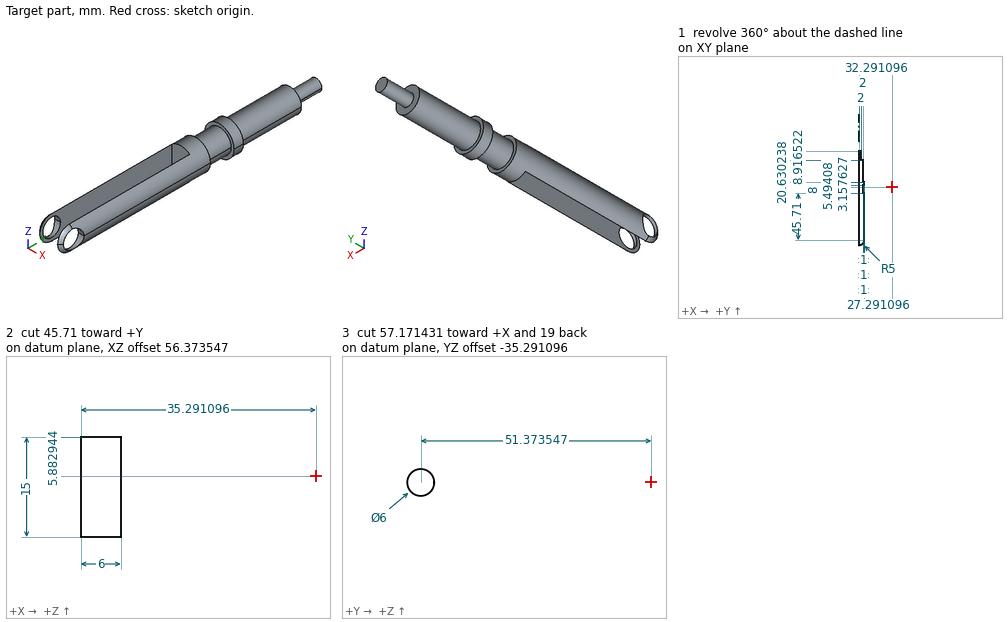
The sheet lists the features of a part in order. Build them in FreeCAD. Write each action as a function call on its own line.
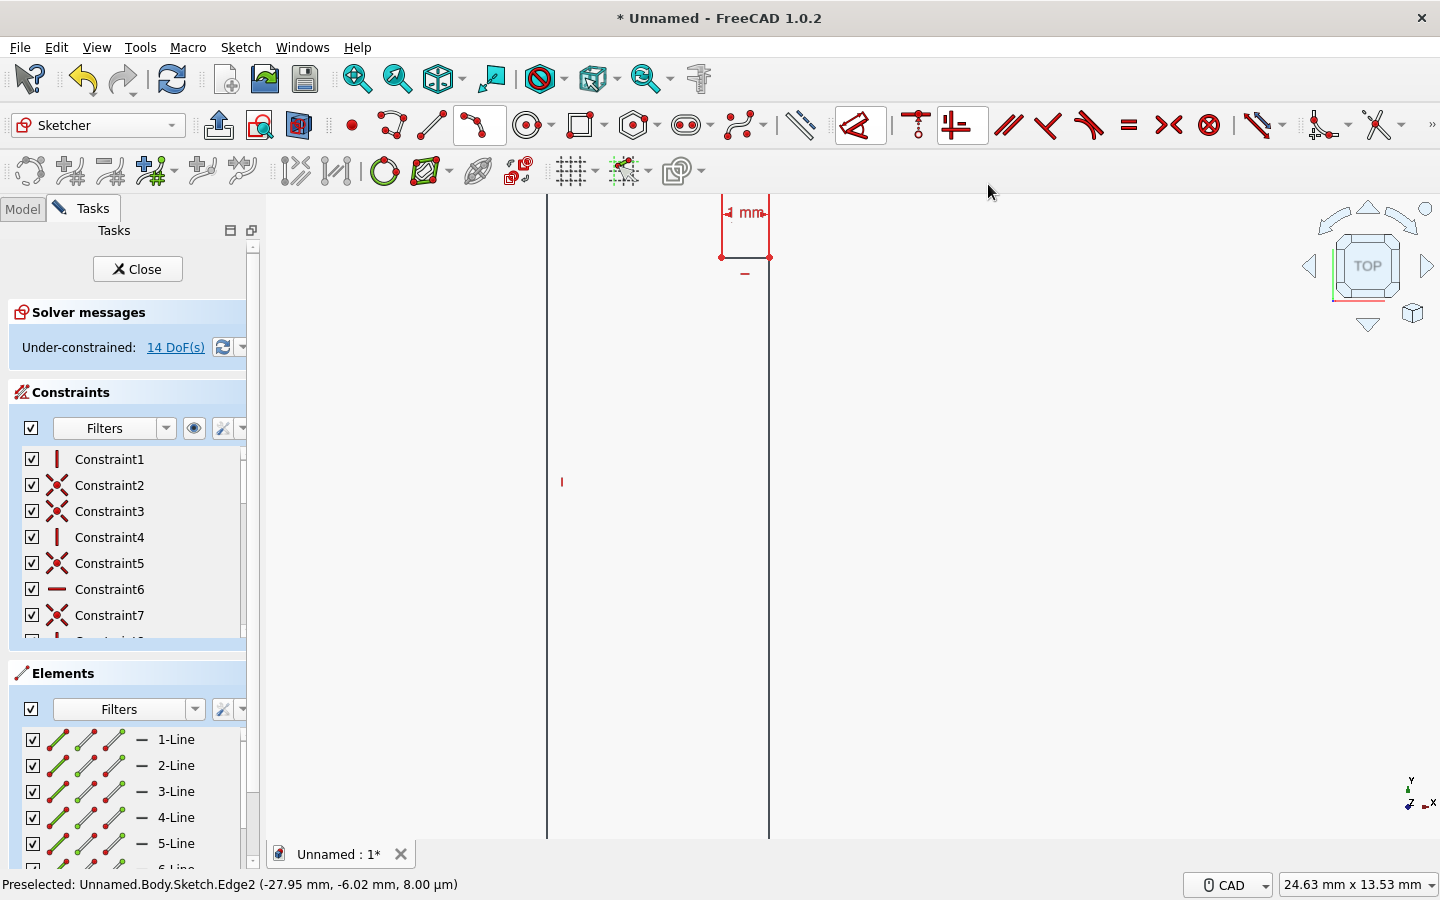
scroll(742, 589, down, 13)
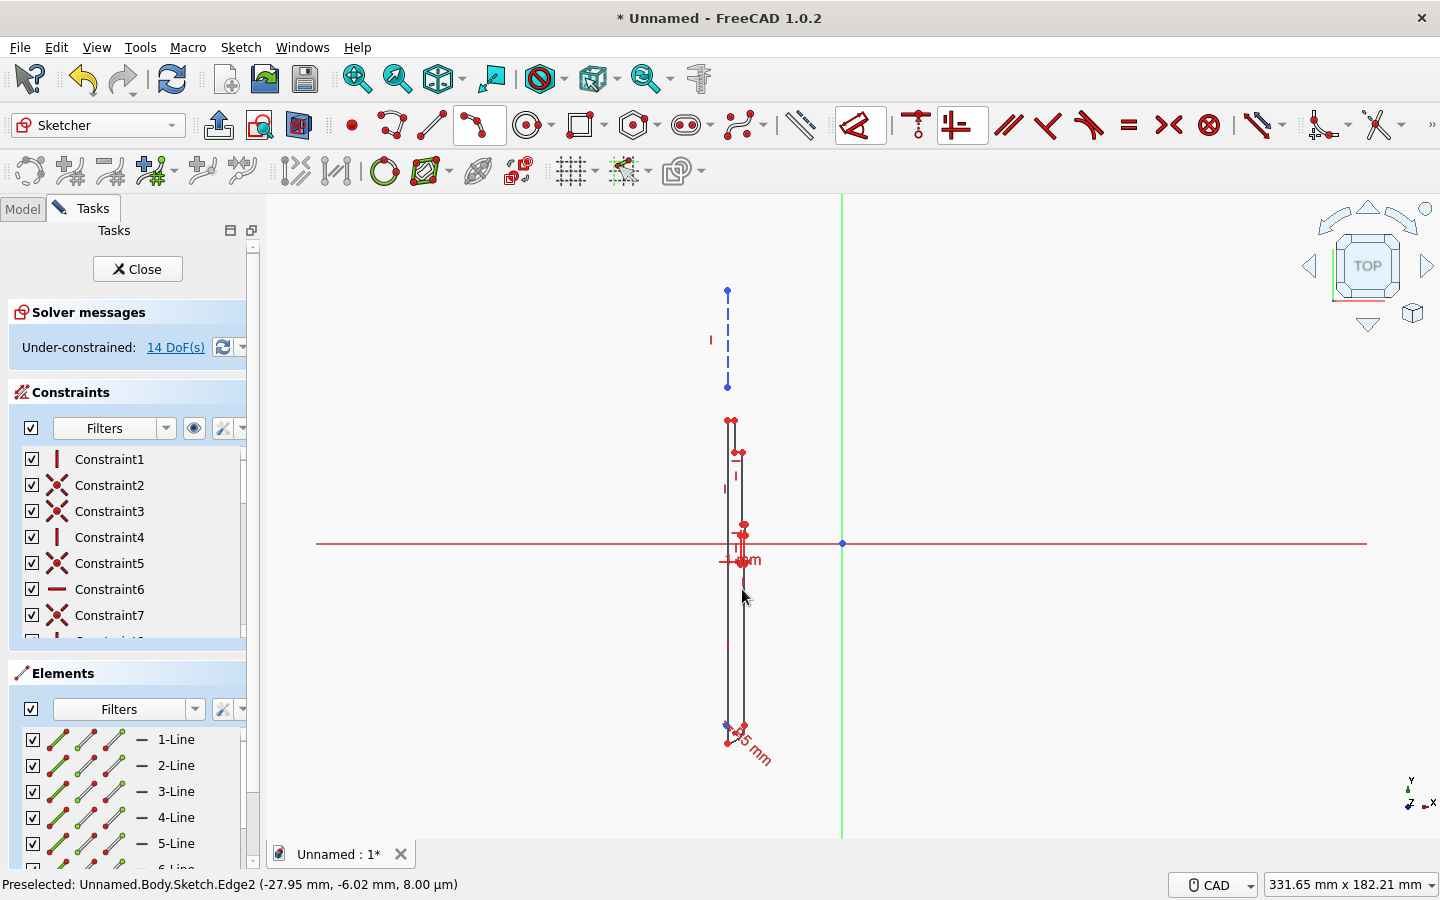
scroll(741, 556, up, 3)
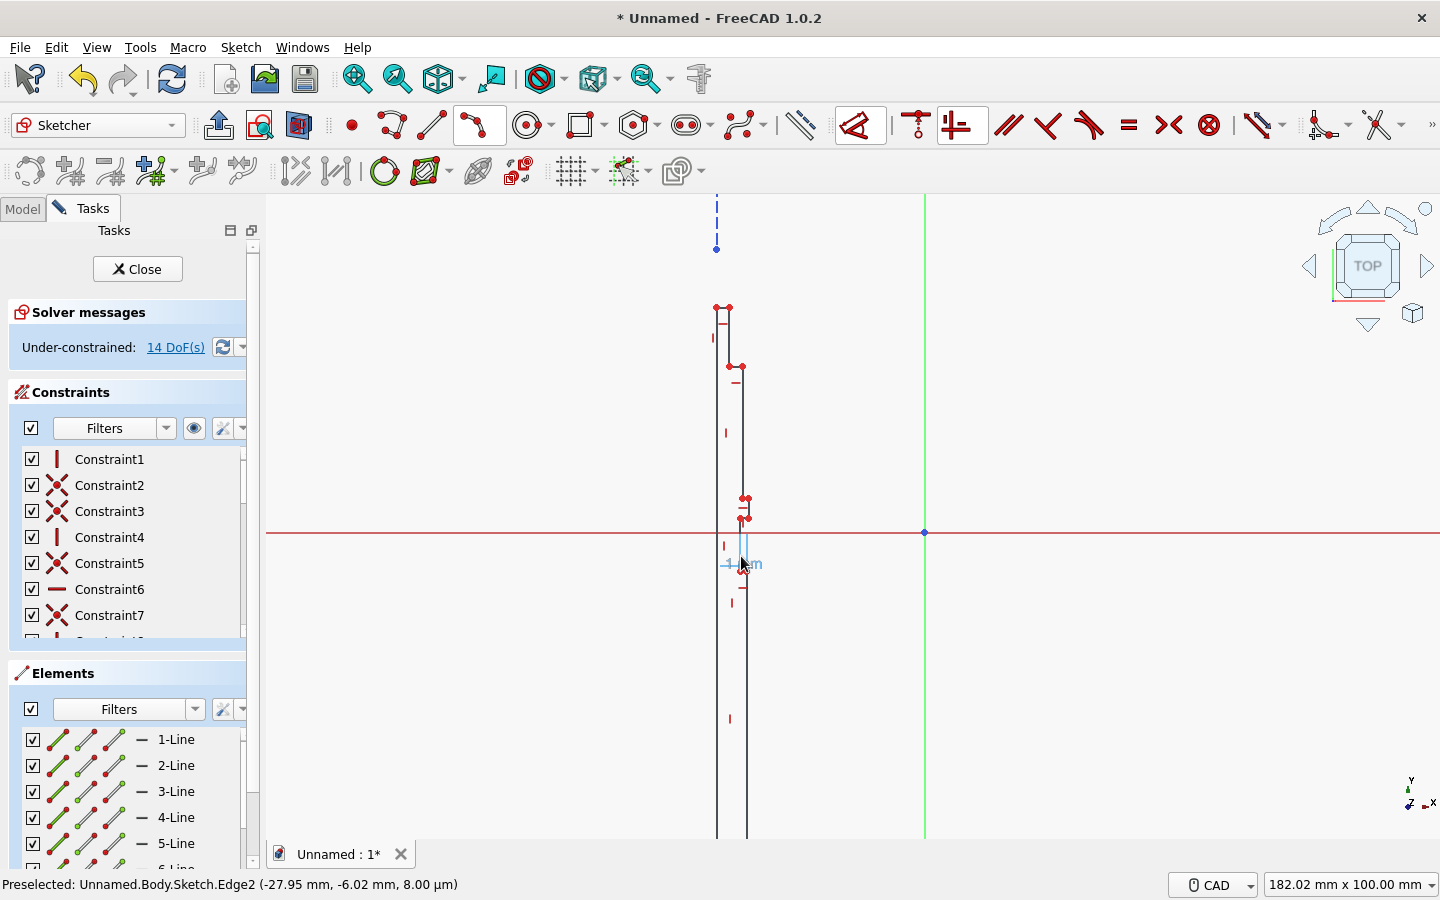
click(740, 556)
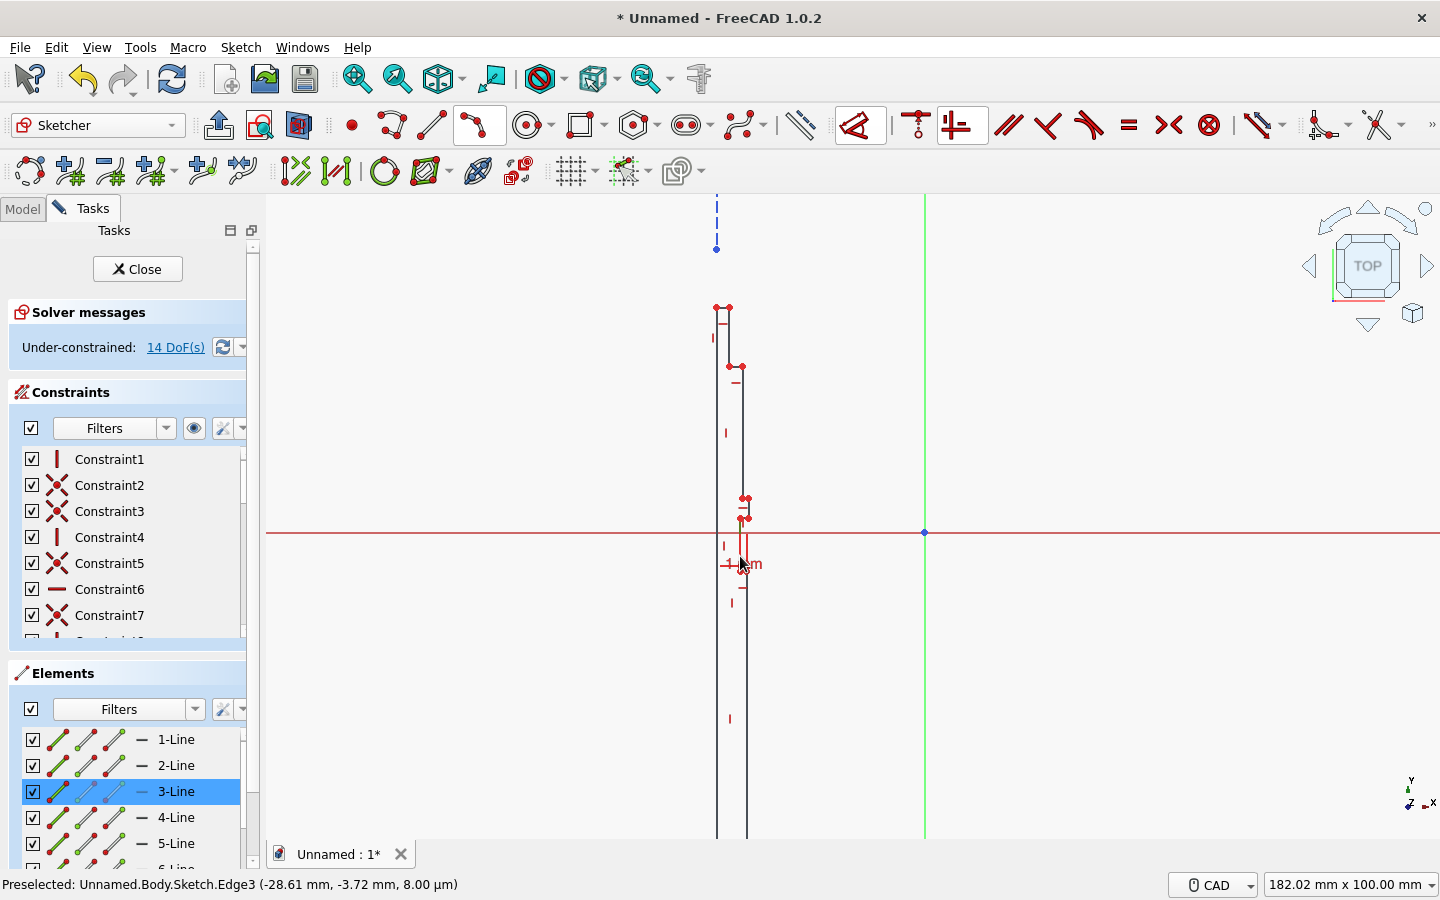
click(880, 126)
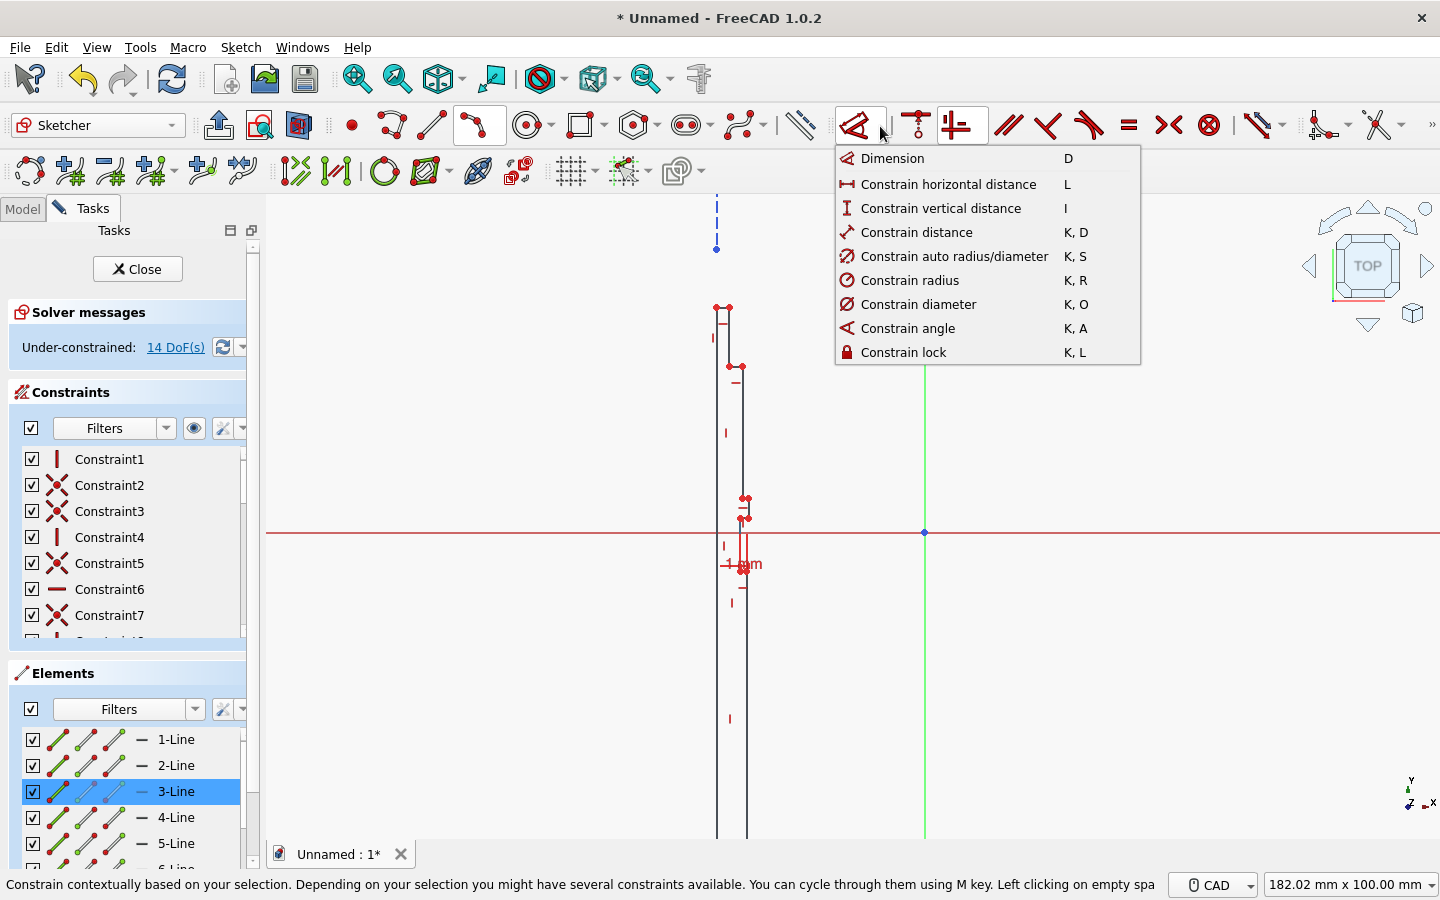
click(988, 208)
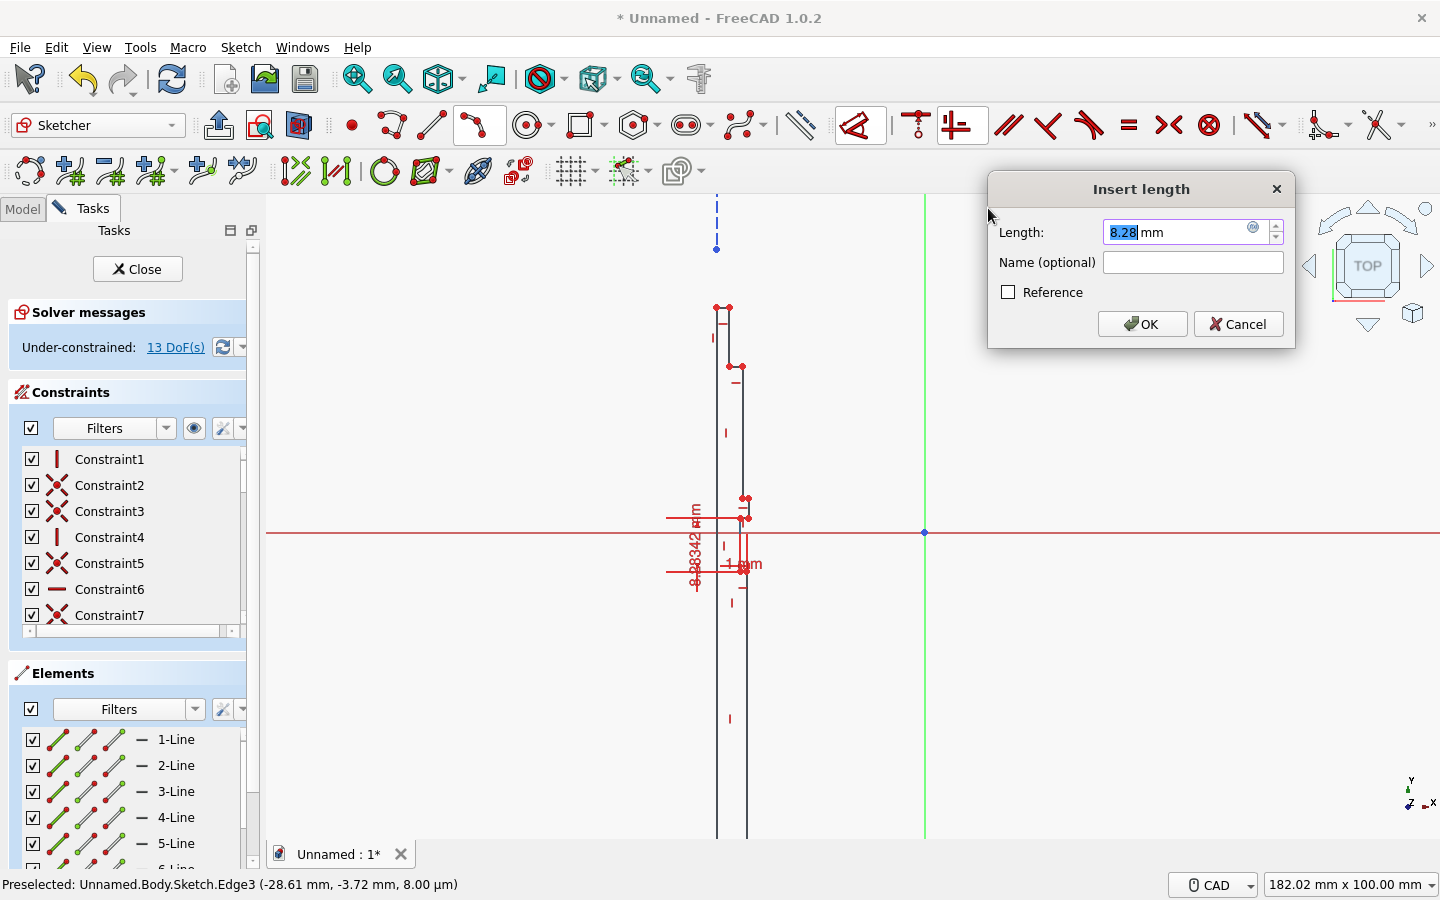
text(8)
key(Return)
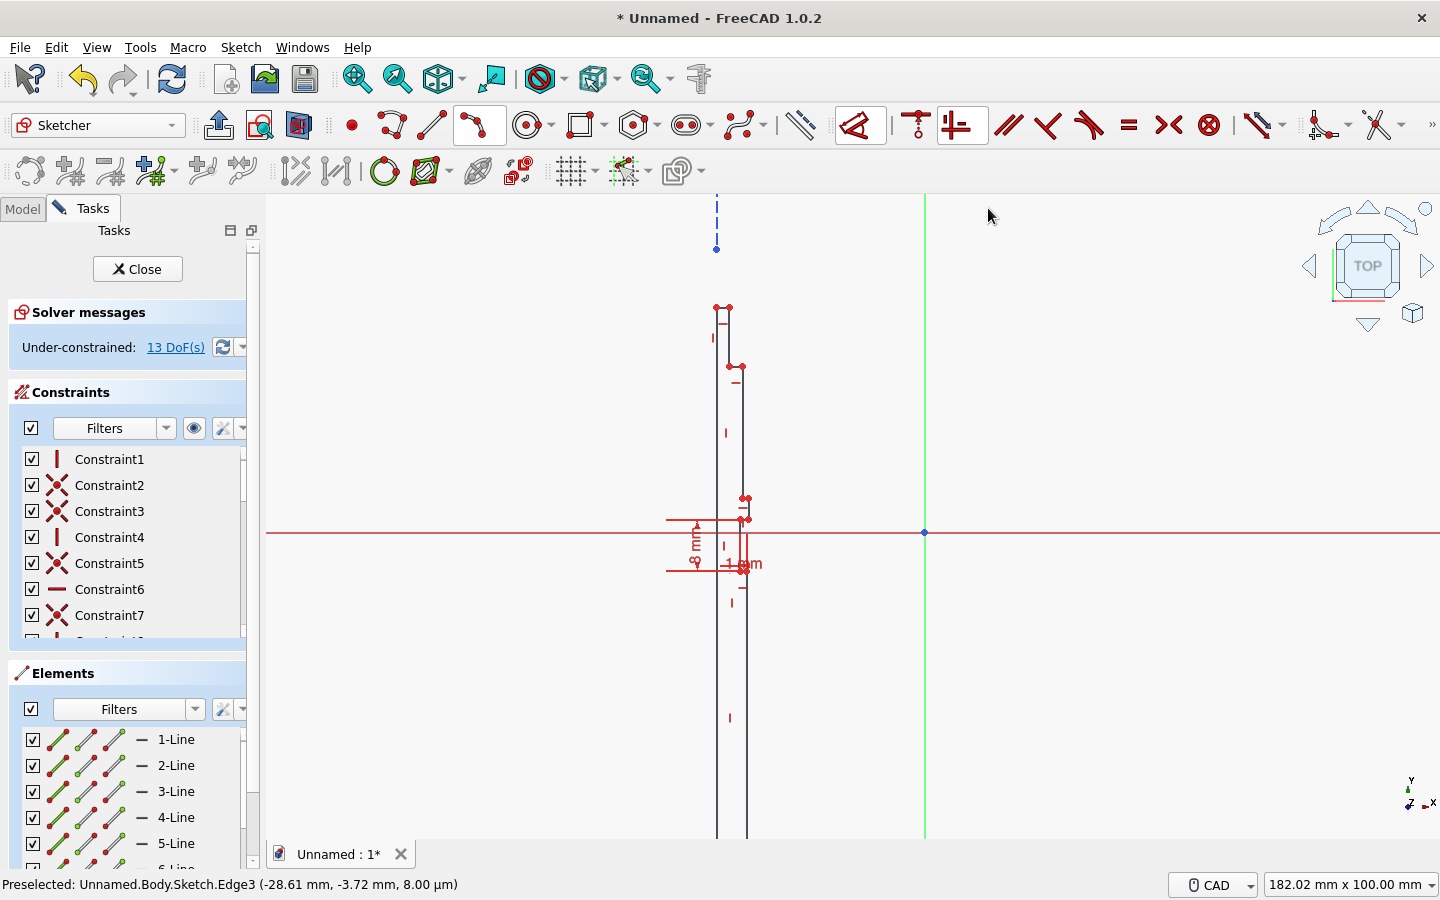
scroll(745, 520, up, 10)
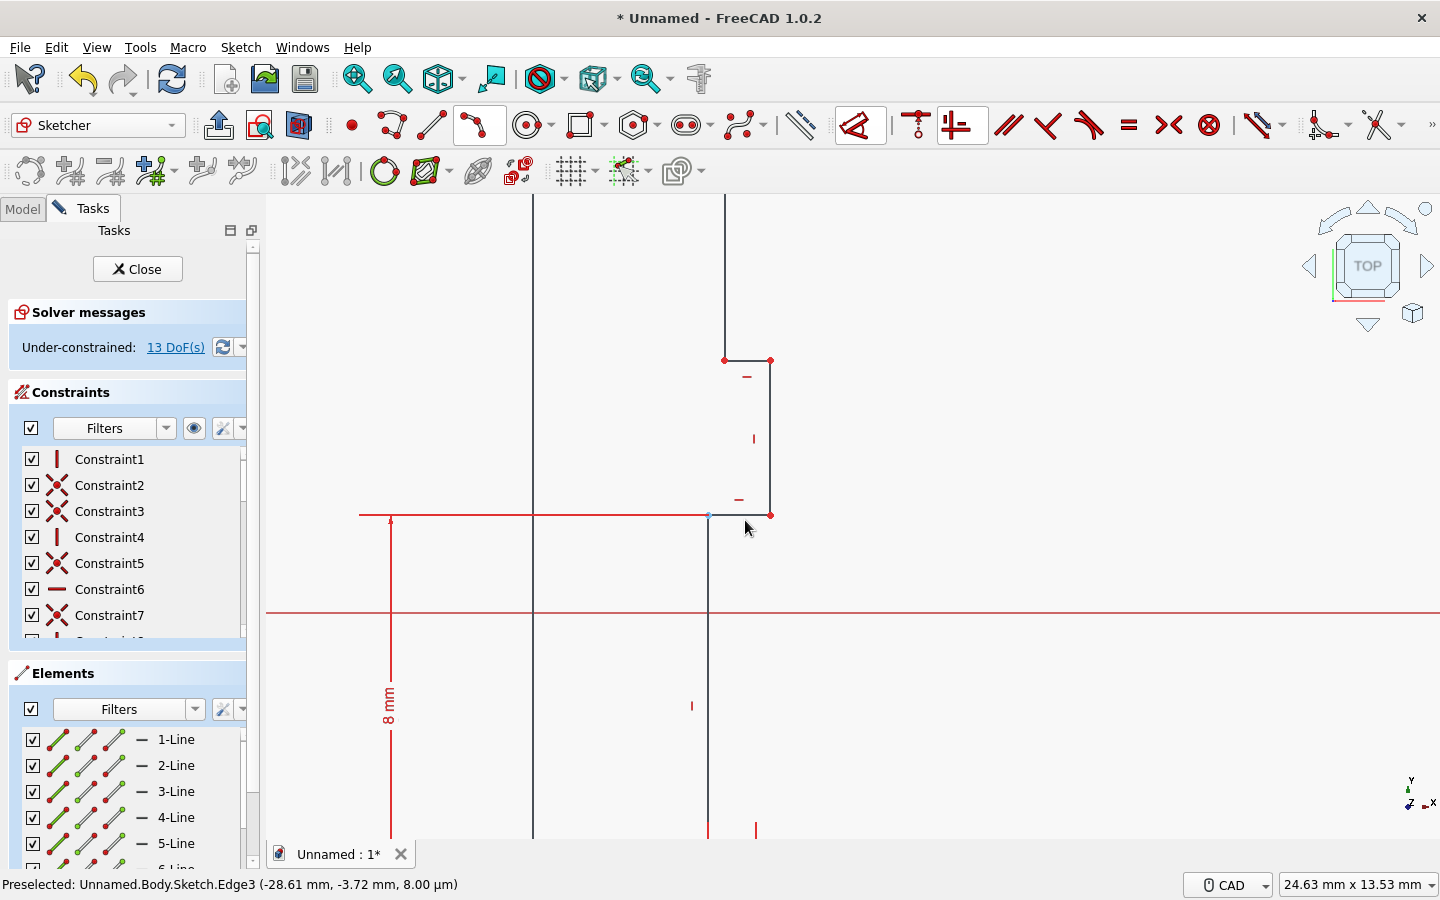
click(739, 515)